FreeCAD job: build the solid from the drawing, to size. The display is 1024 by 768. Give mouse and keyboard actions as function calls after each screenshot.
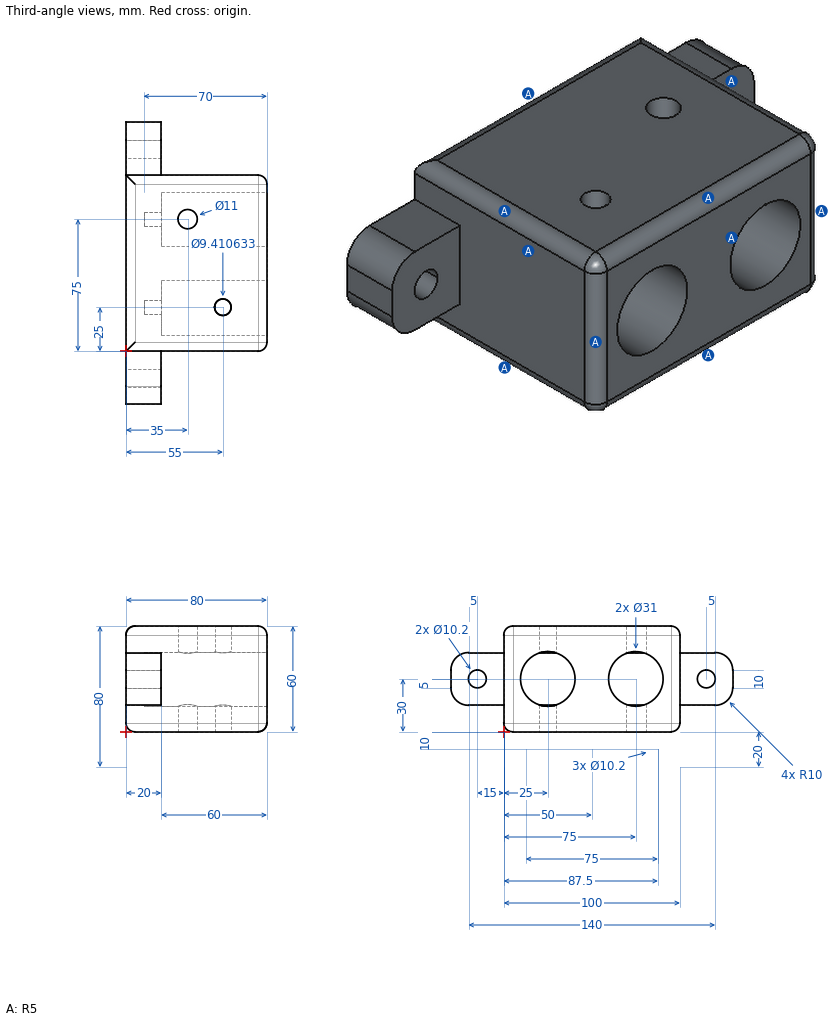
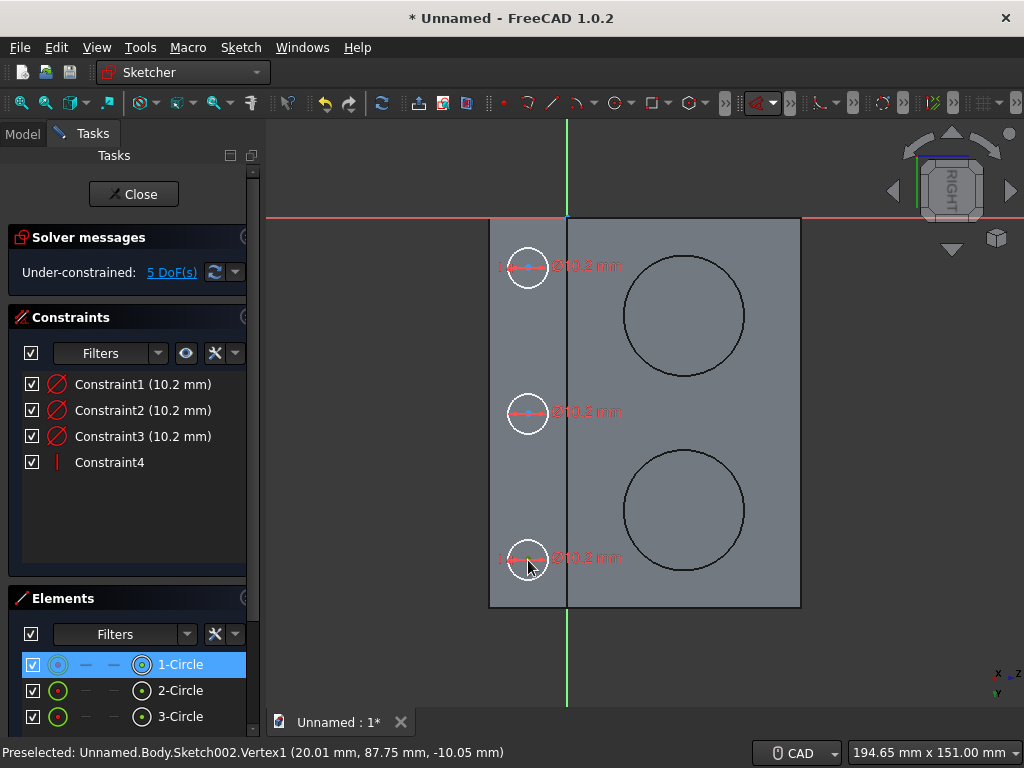
click(528, 414)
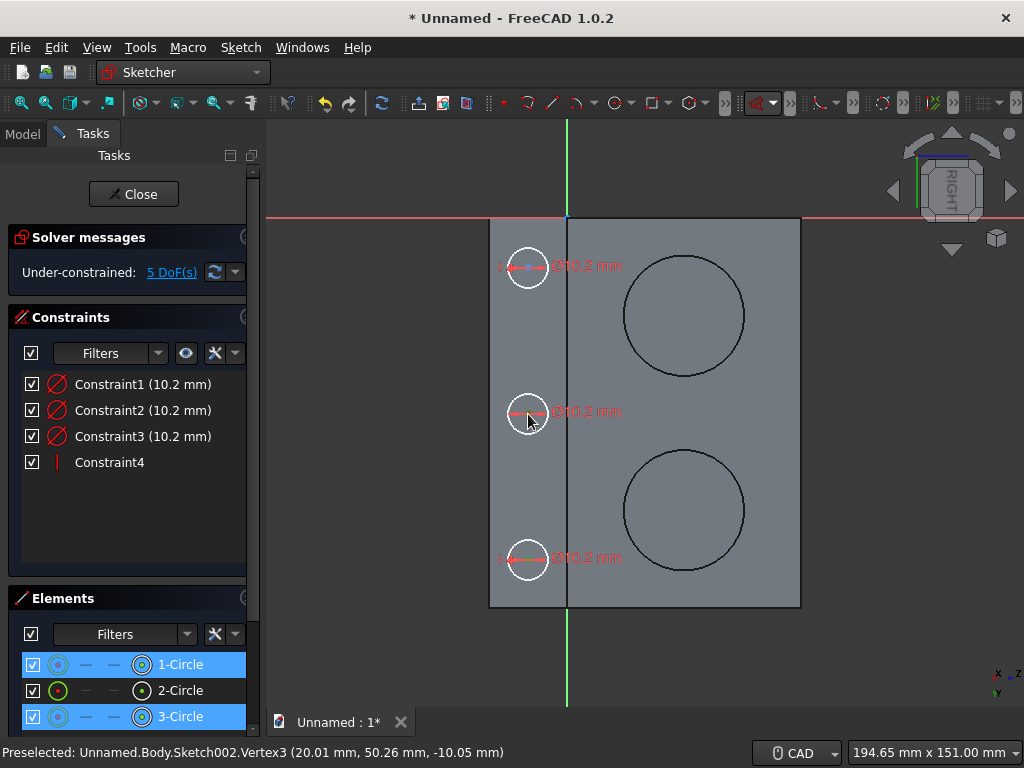
key(v)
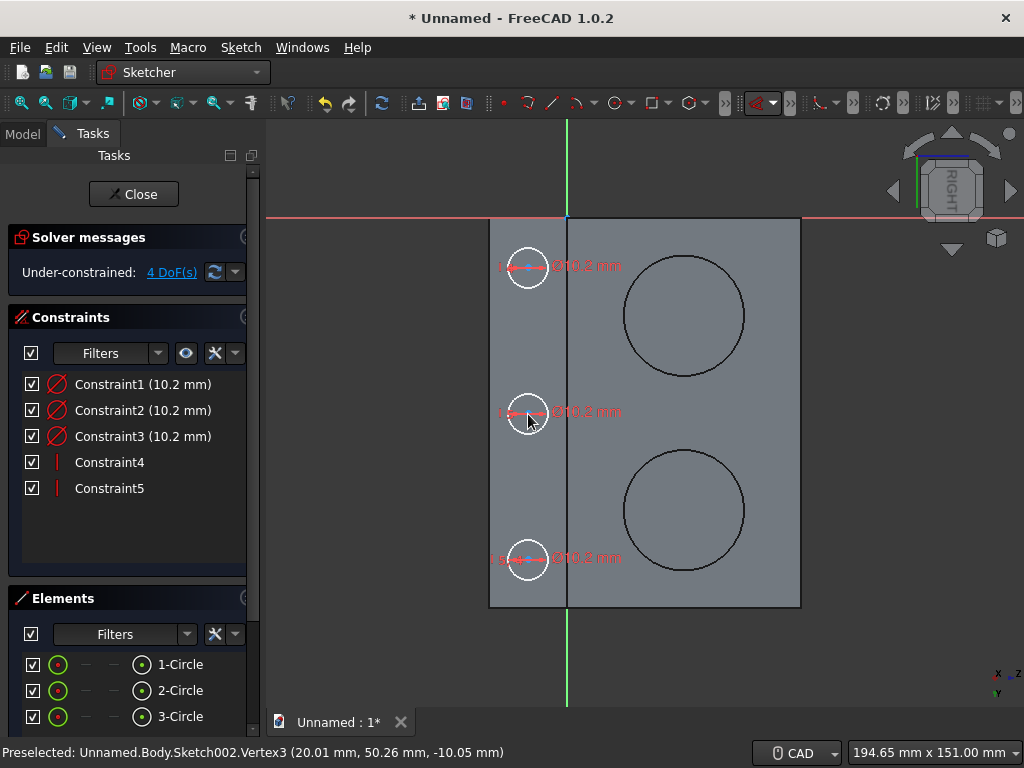
click(528, 560)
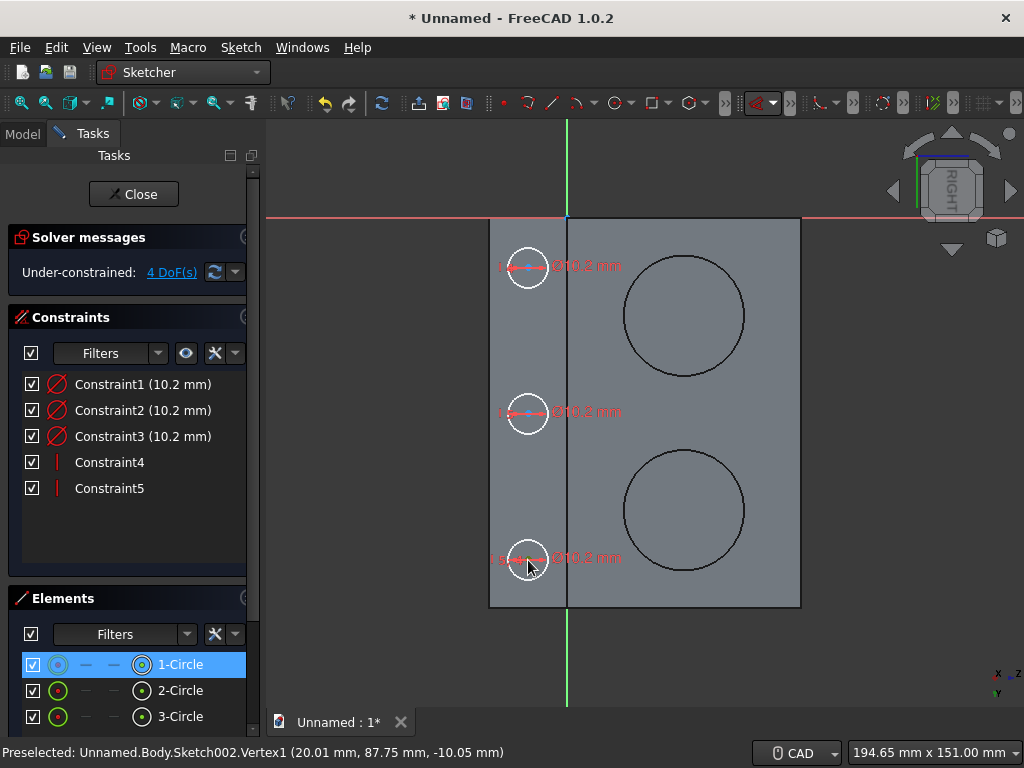
key(l)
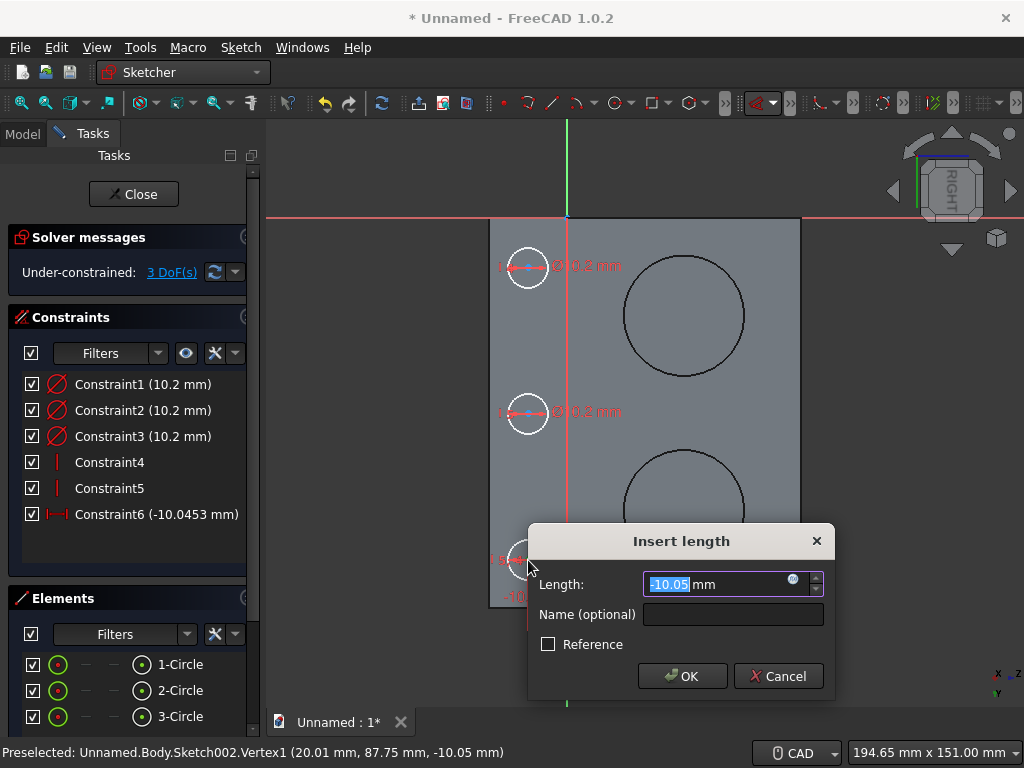
text(-10)
key(Return)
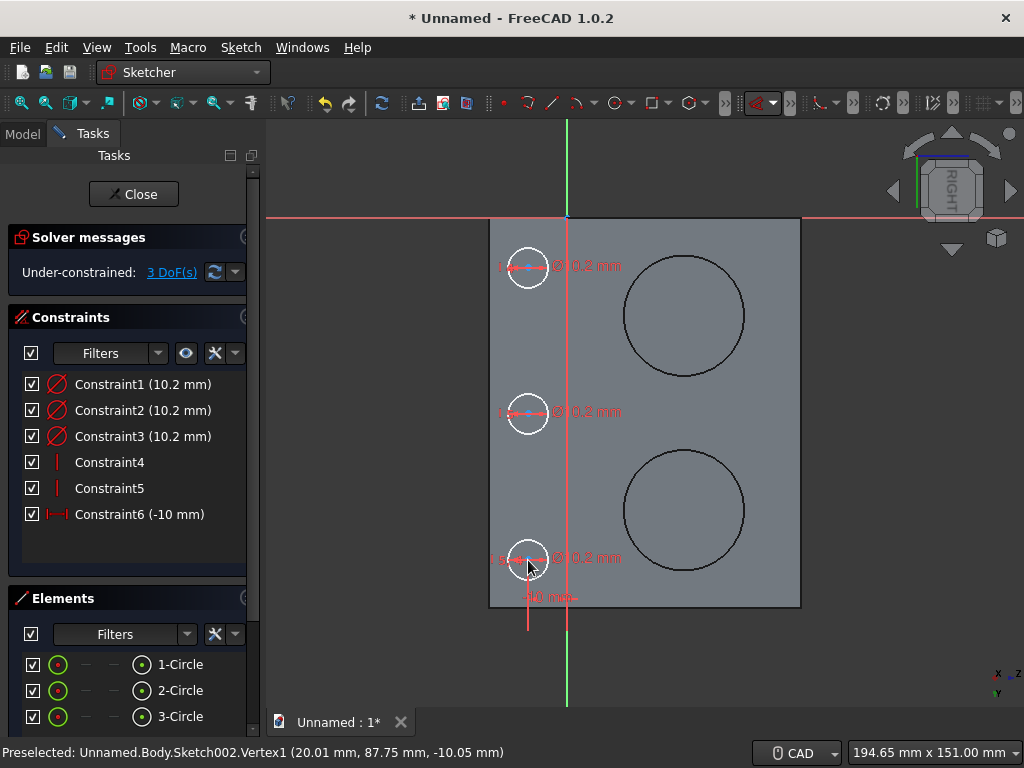
click(528, 414)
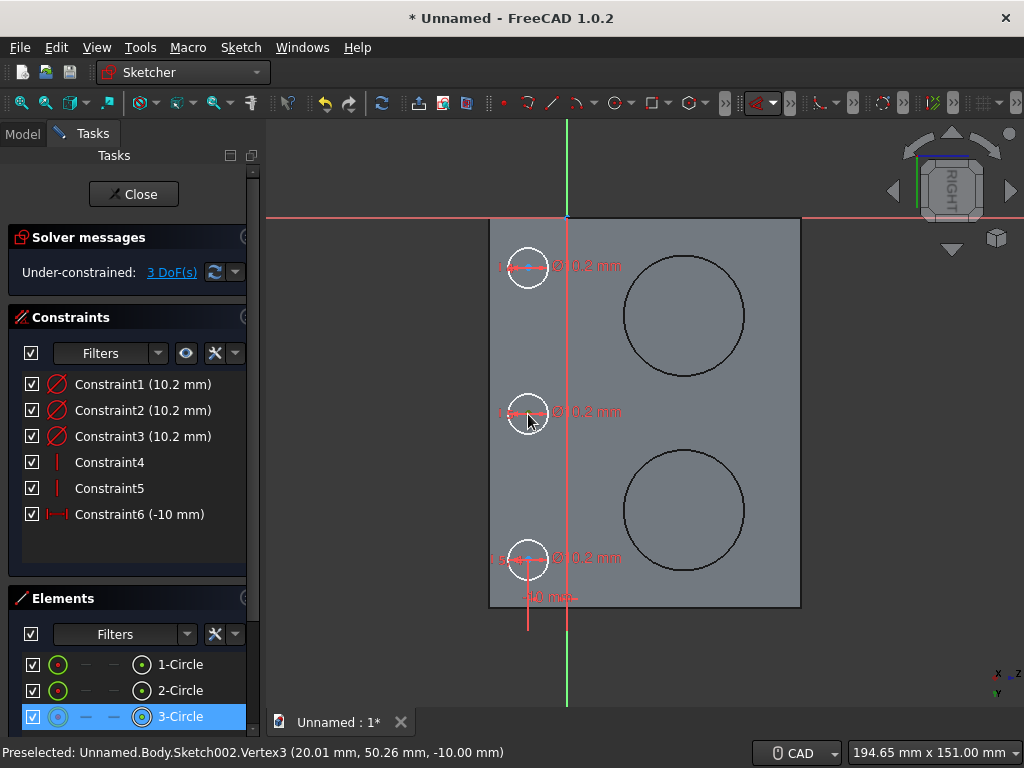
key(i)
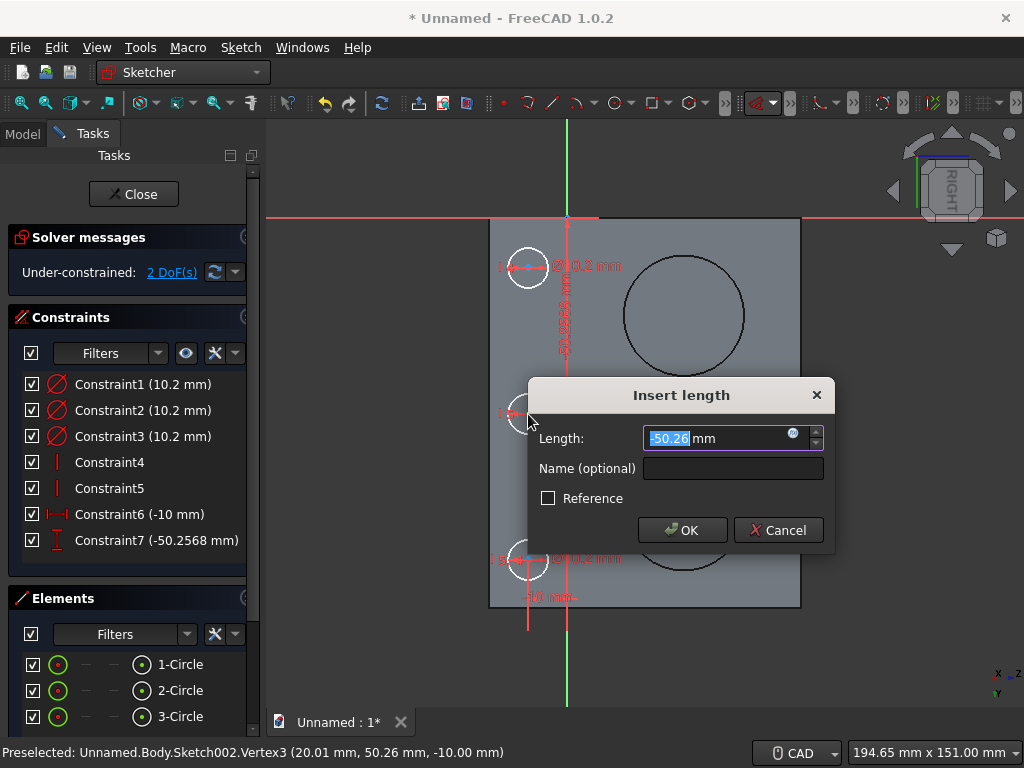
text(-50)
key(Return)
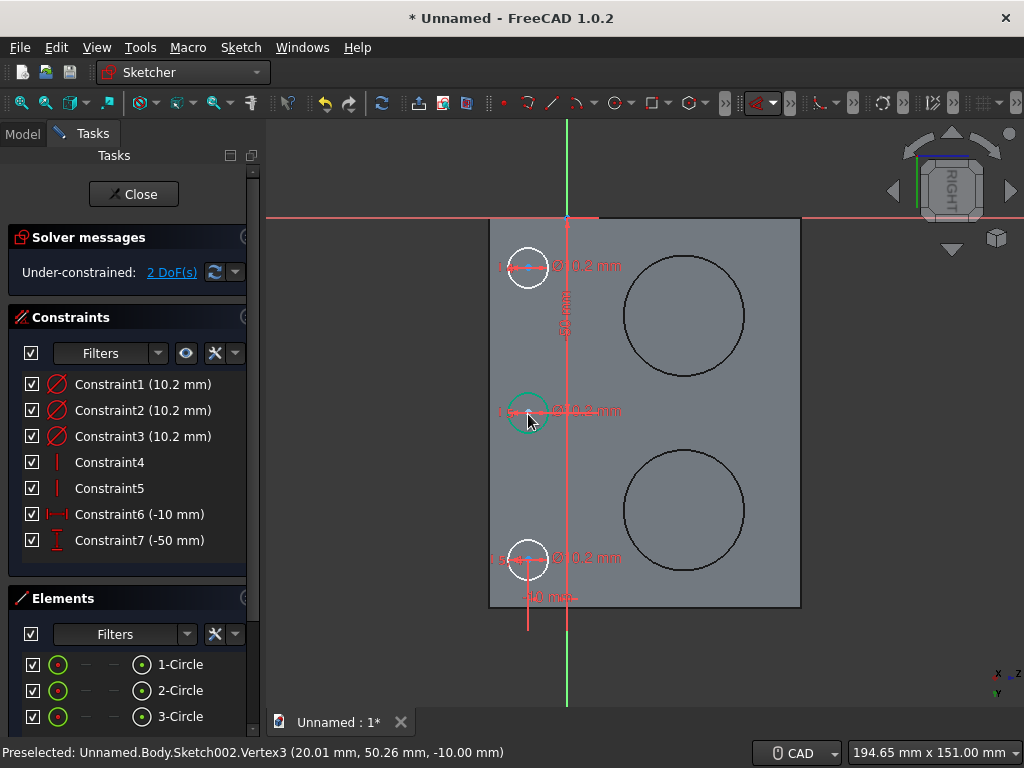
click(528, 560)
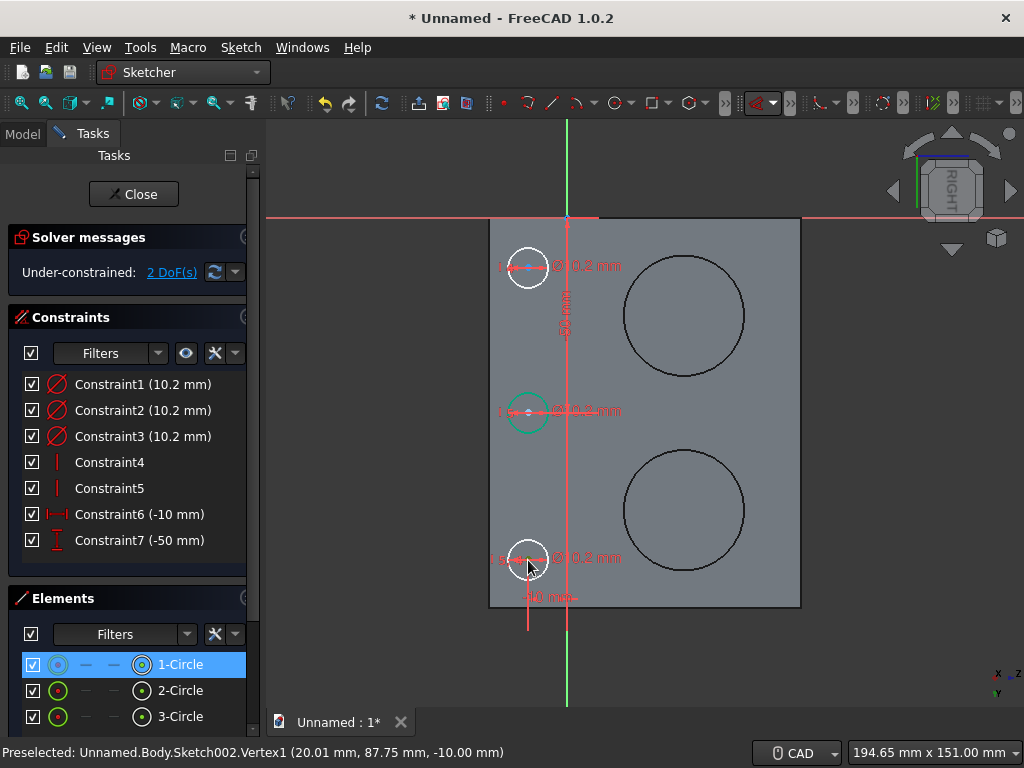
click(528, 268)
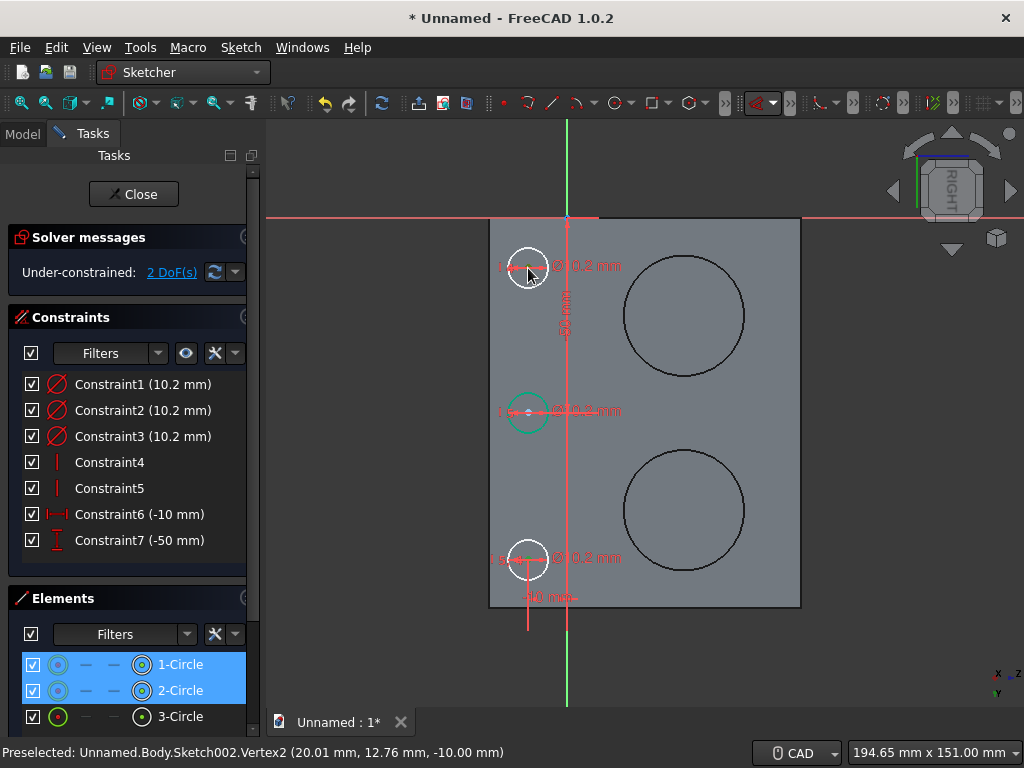
key(i)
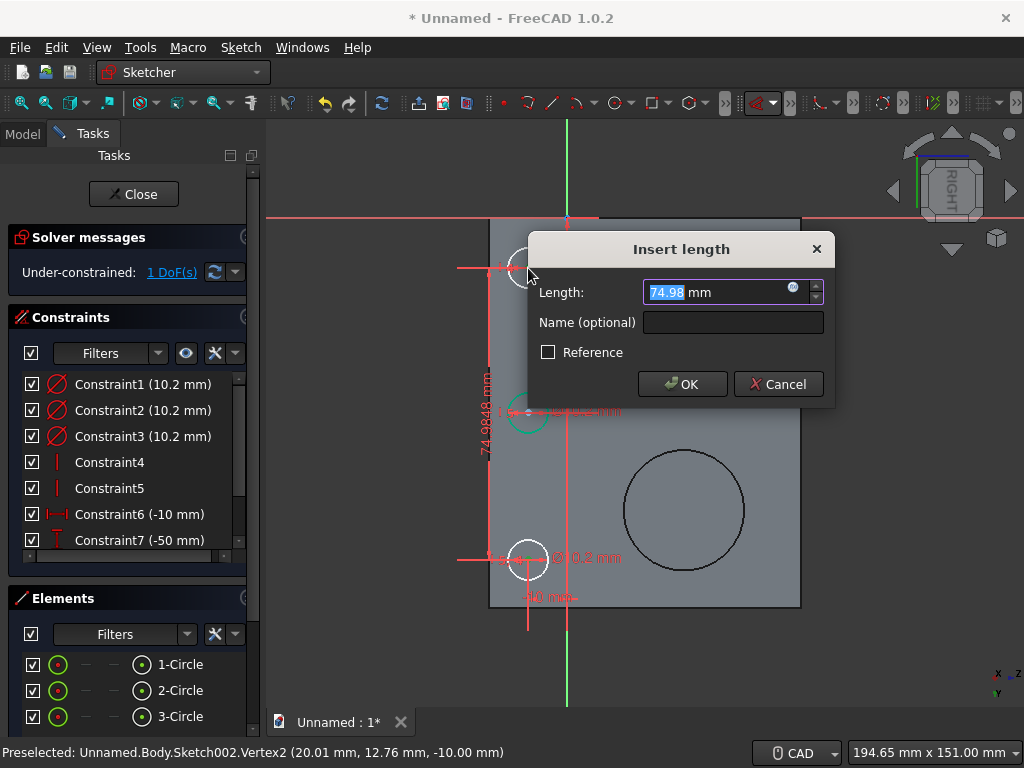
text(75)
key(Return)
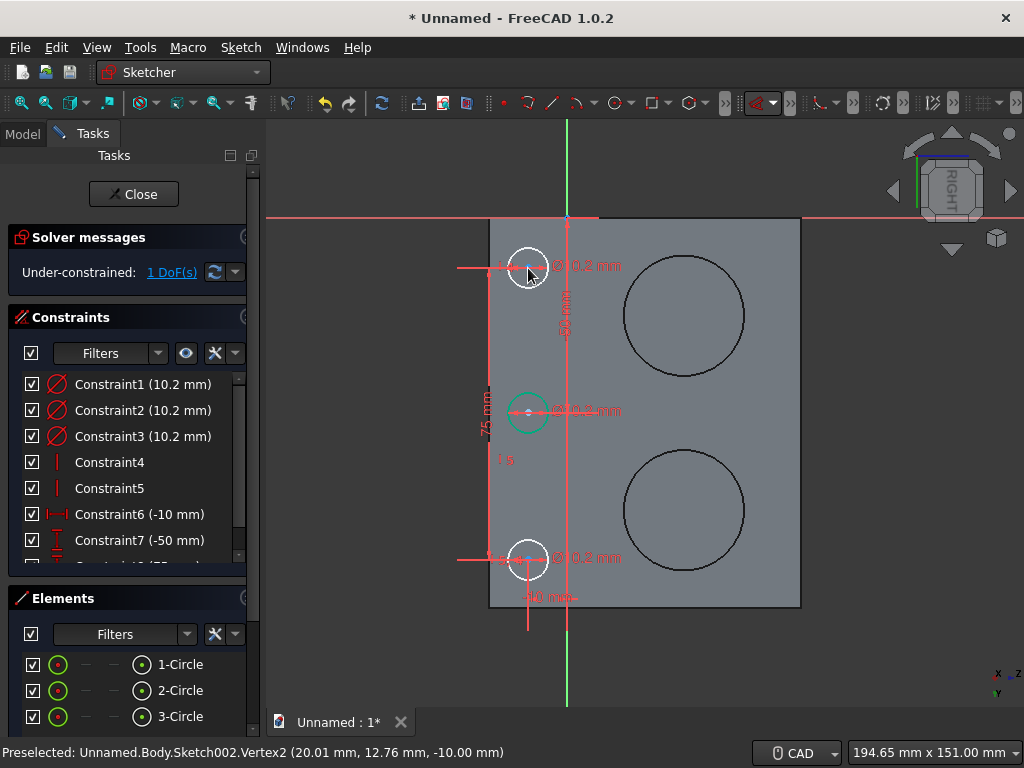
click(528, 560)